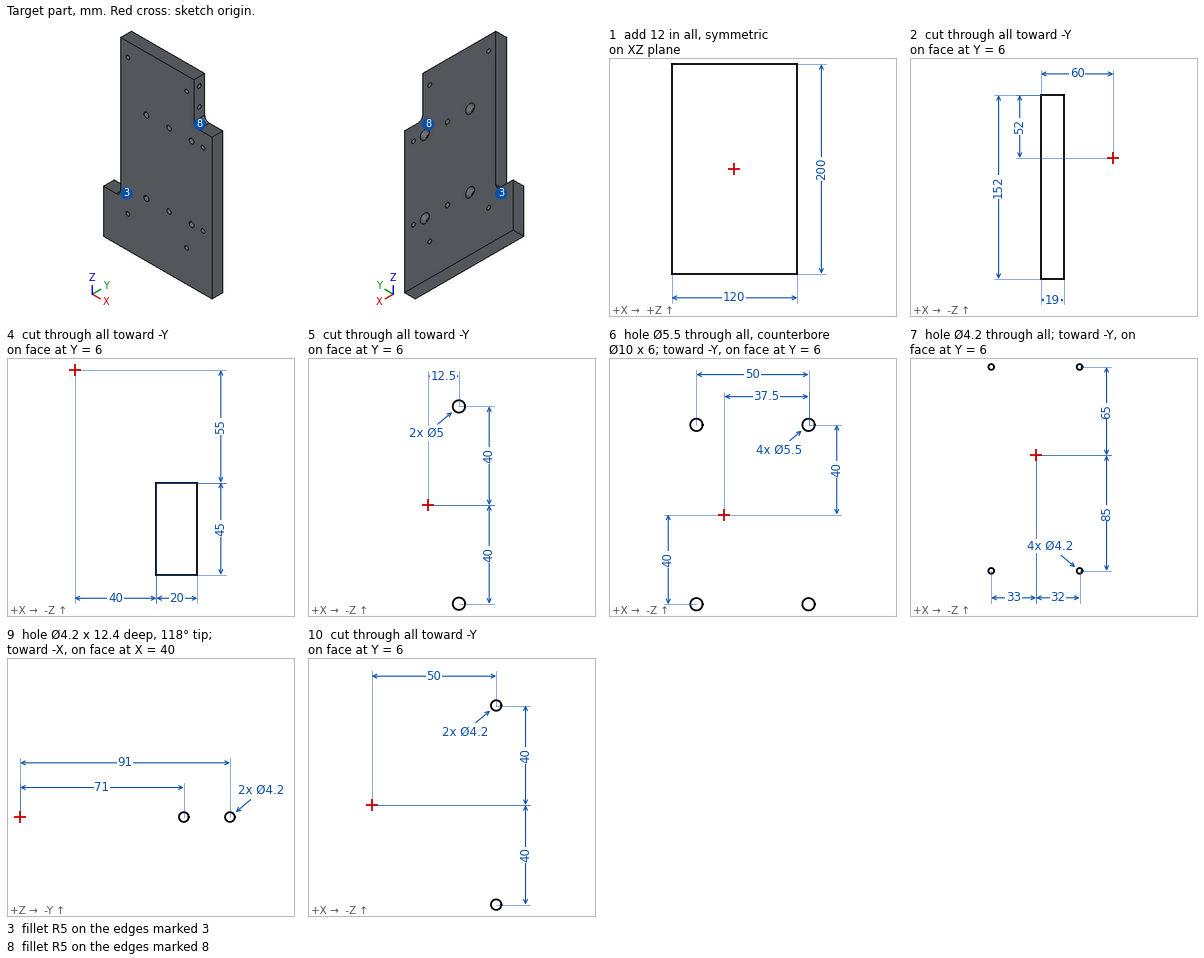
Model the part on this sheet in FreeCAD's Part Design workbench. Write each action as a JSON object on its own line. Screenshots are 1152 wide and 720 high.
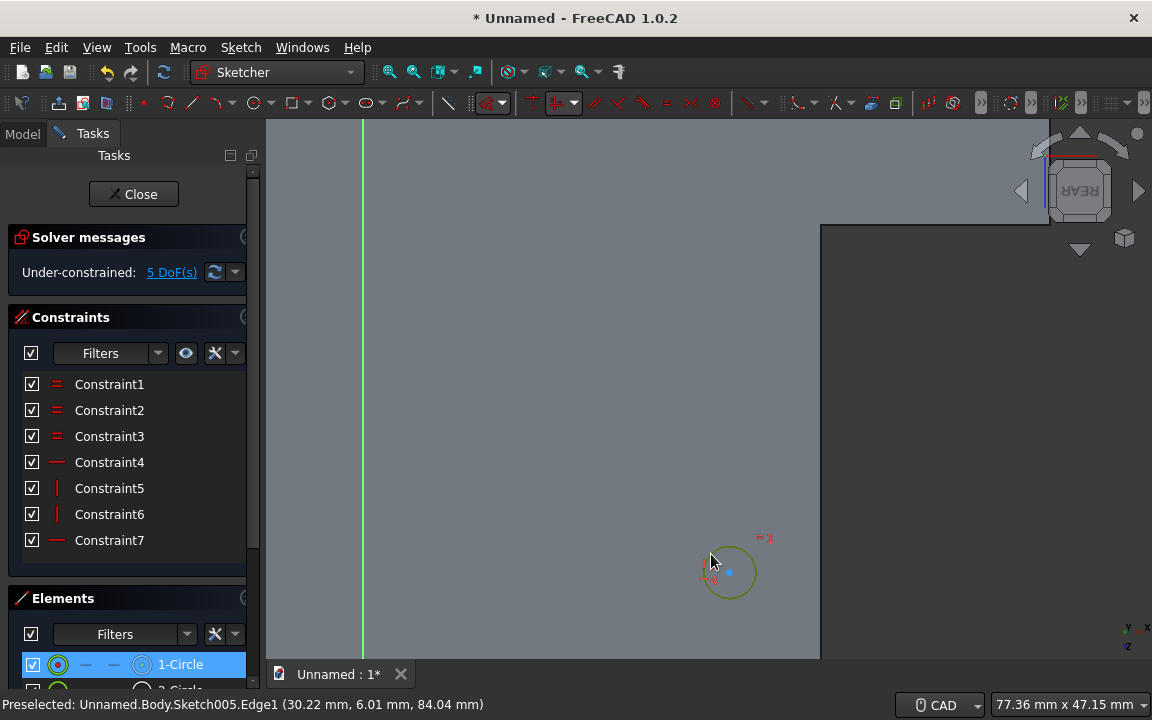
{"action": "left_click", "coordinate": [504, 104]}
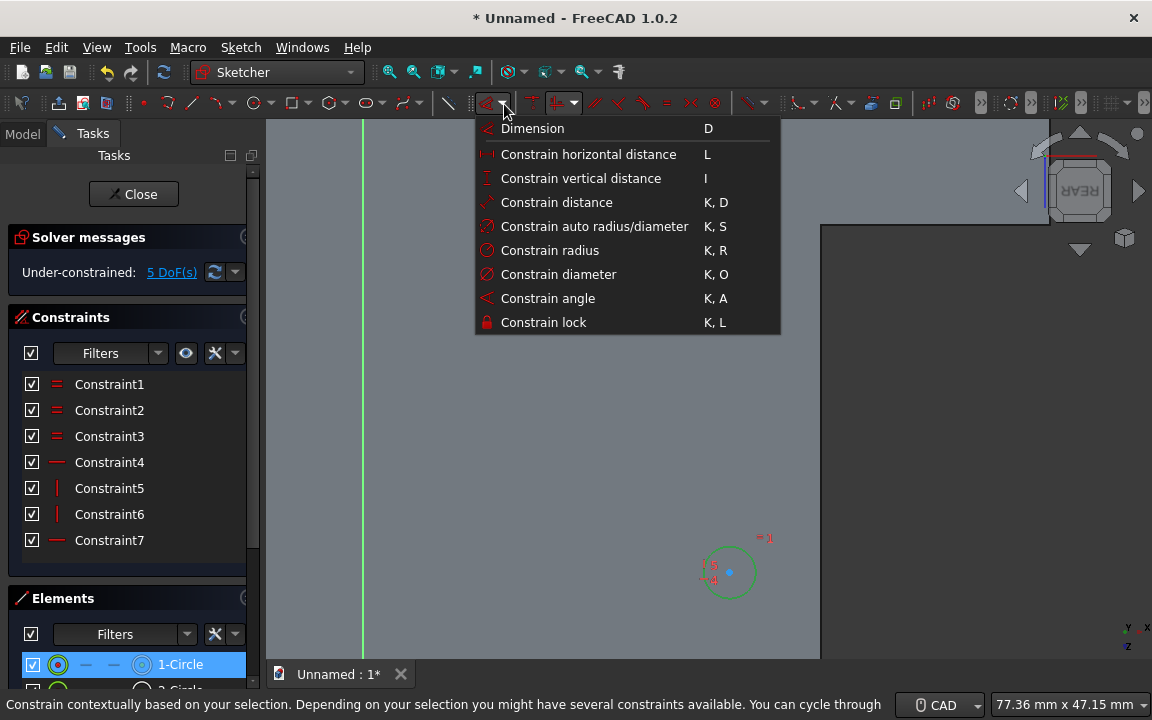
{"action": "left_click", "coordinate": [628, 274]}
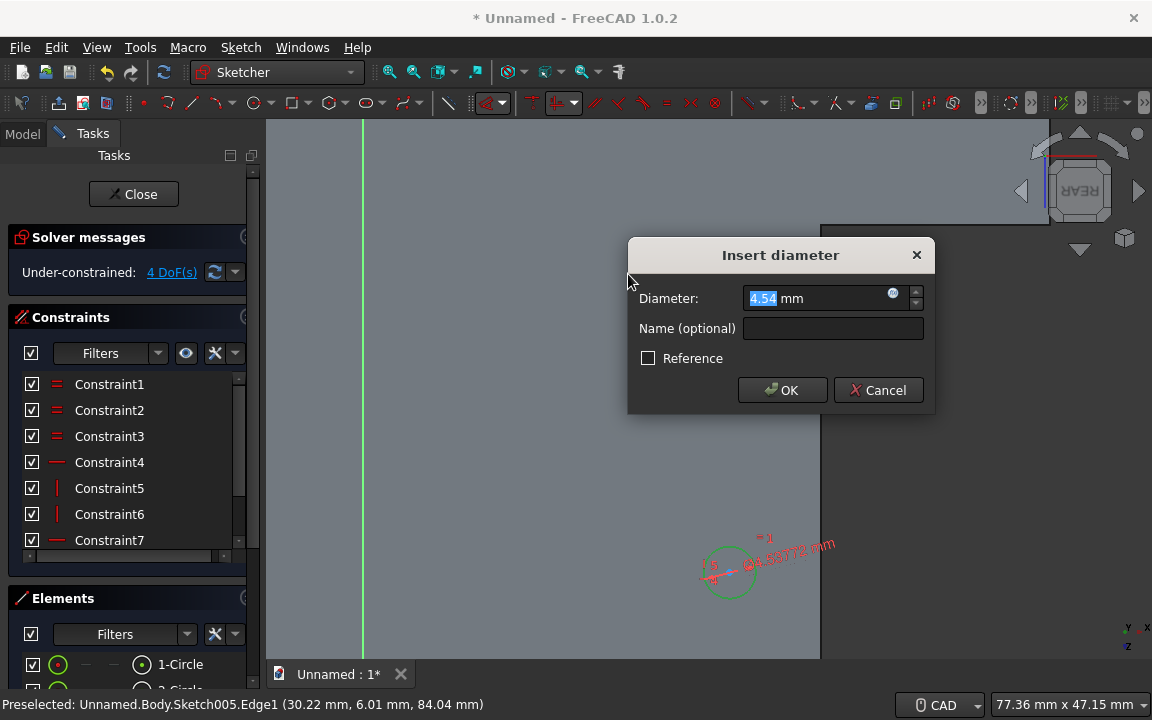
{"action": "type", "text": "4.2"}
{"action": "key", "text": "Return"}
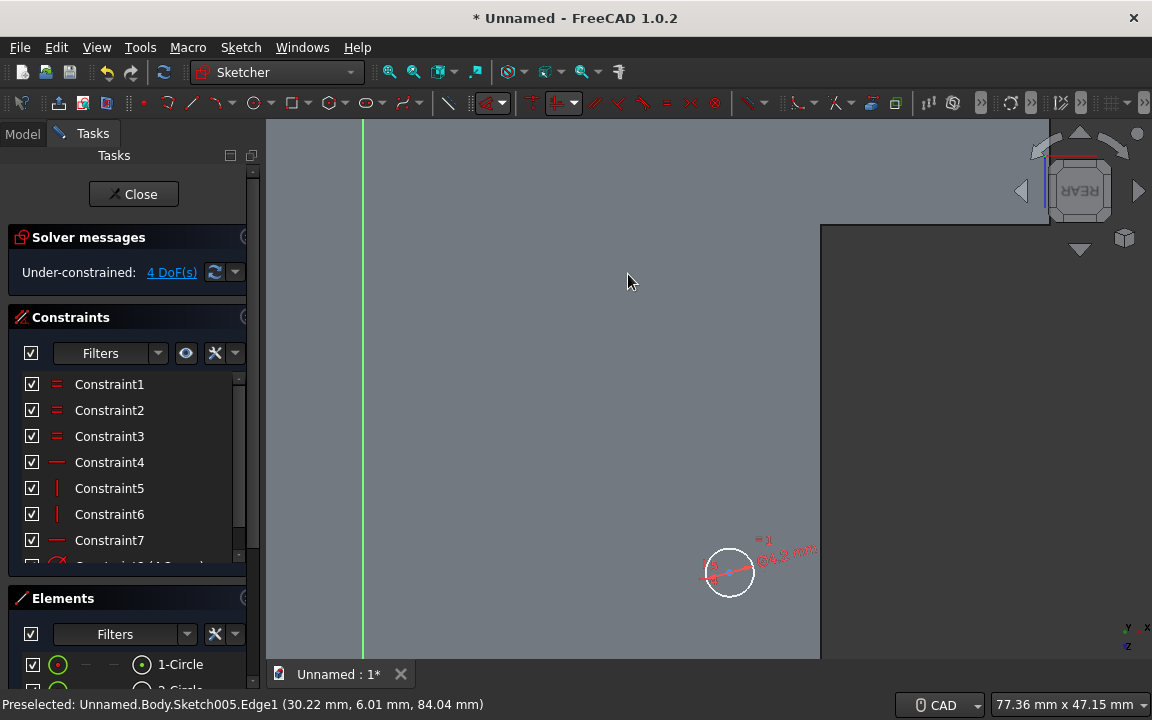
{"action": "scroll", "coordinate": [712, 561], "scroll_direction": "down", "scroll_amount": 8}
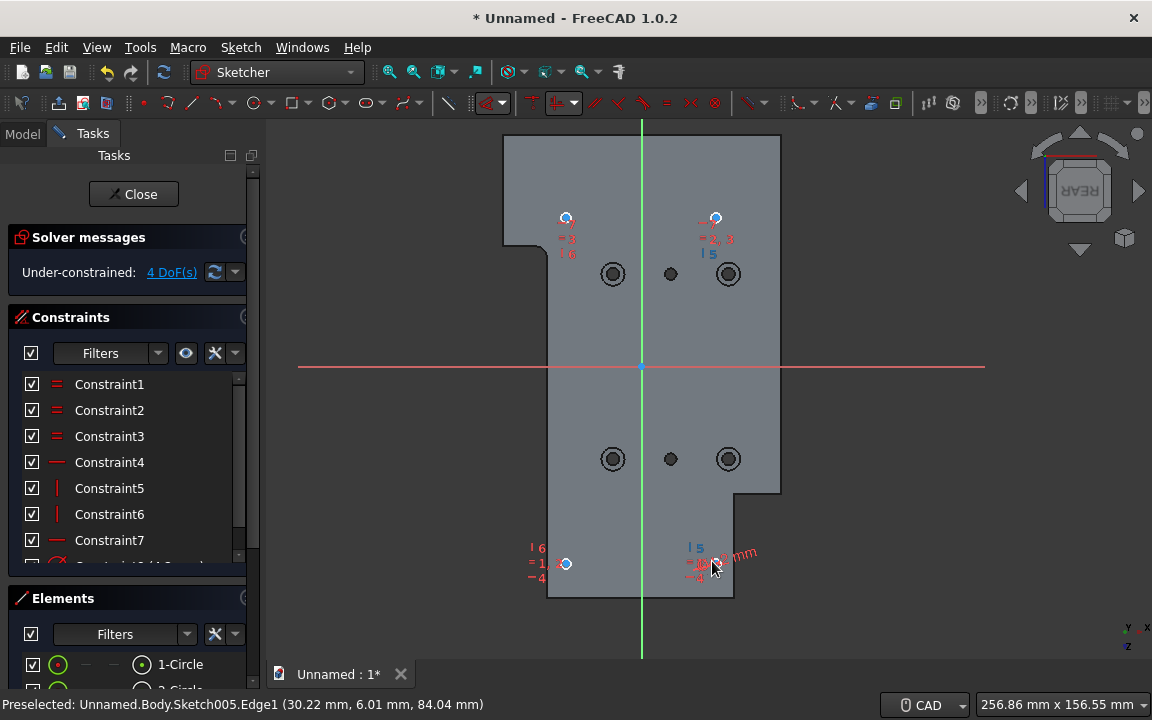
{"action": "left_click", "coordinate": [716, 564]}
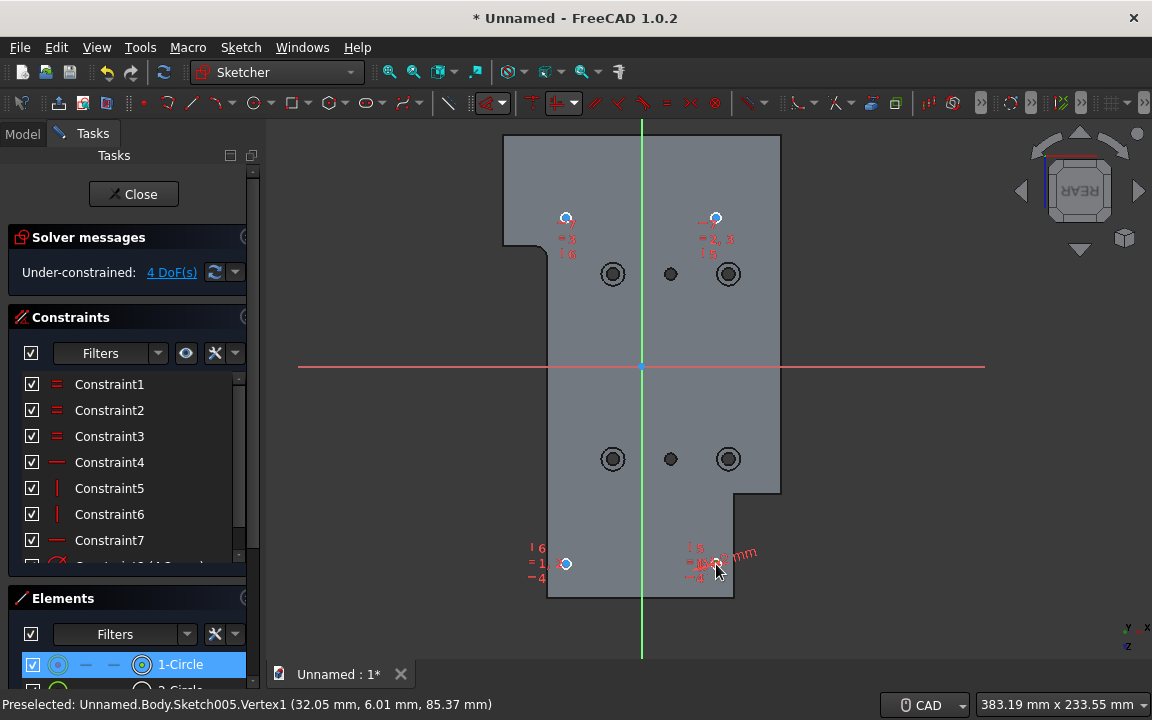
{"action": "left_click", "coordinate": [504, 104]}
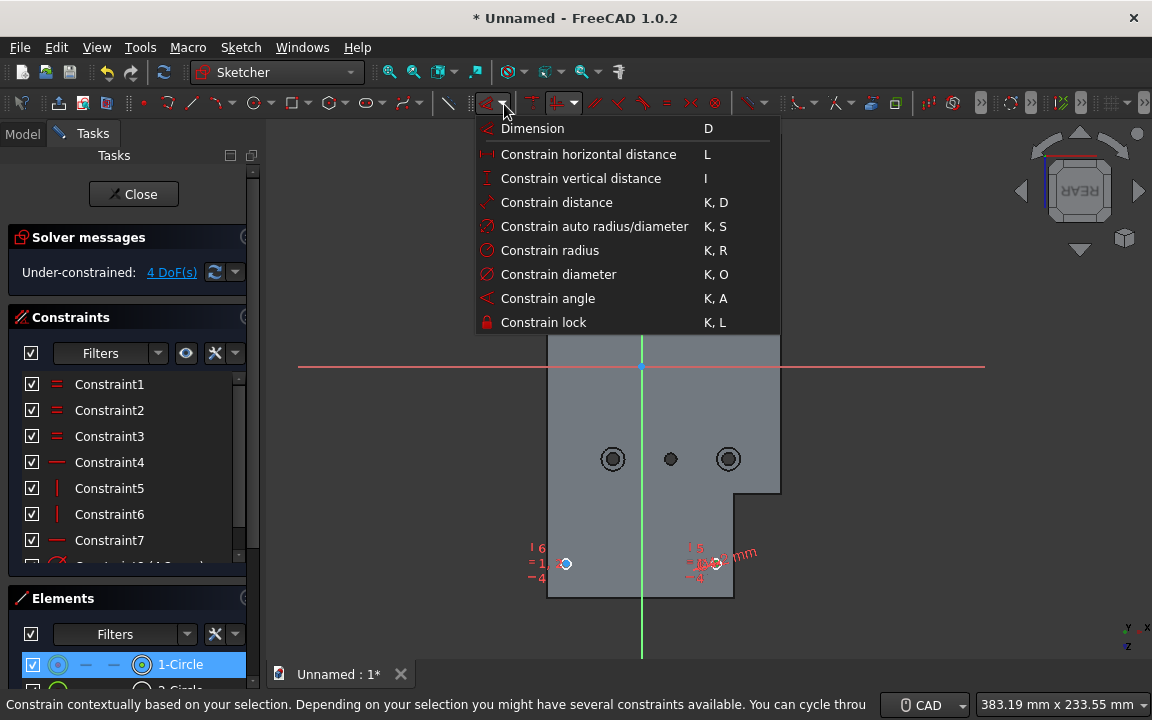
{"action": "left_click", "coordinate": [628, 154]}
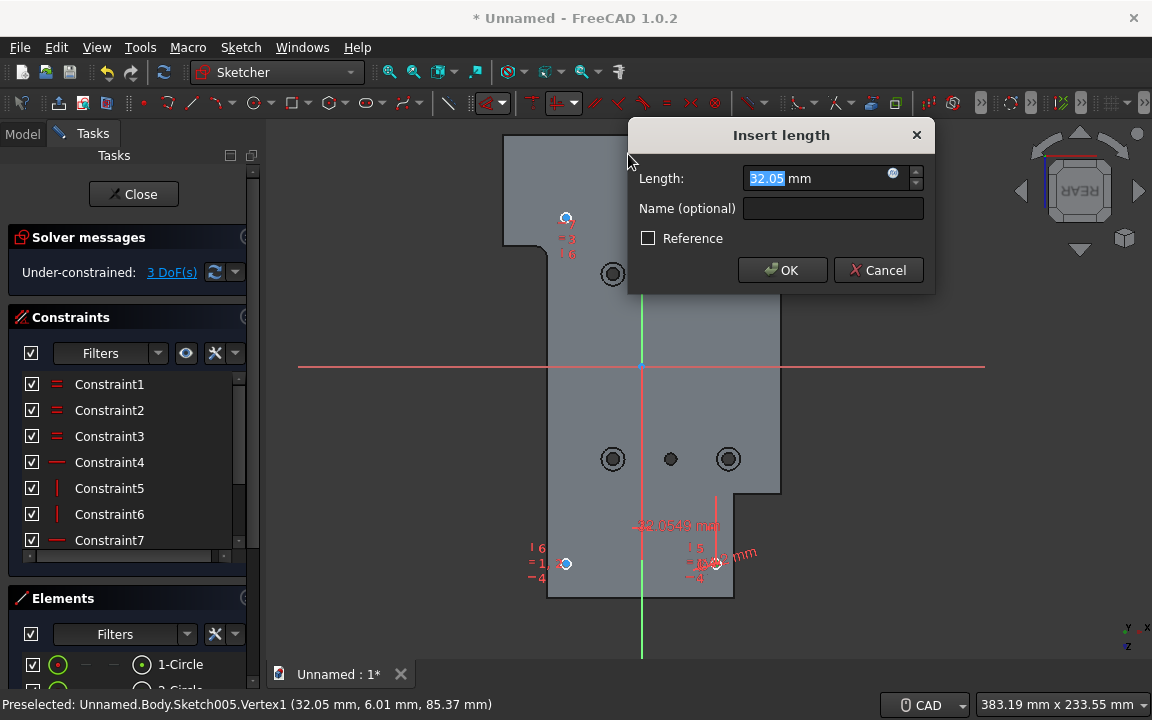
{"action": "type", "text": "32"}
{"action": "key", "text": "Return"}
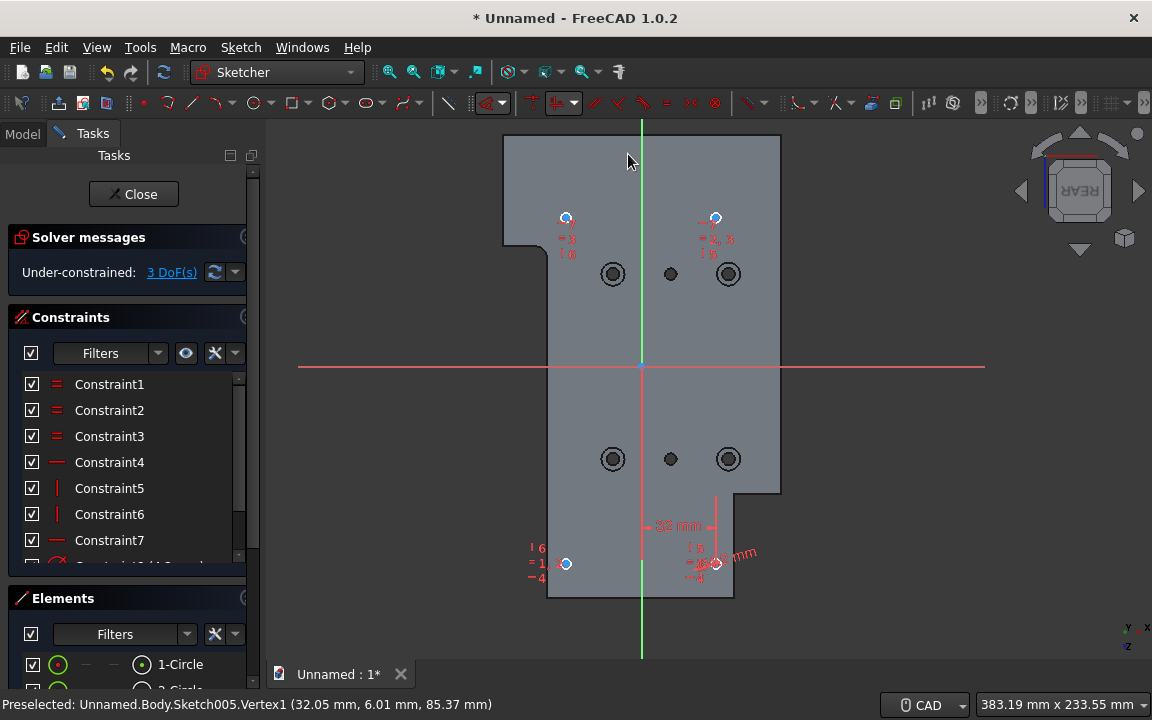
{"action": "left_click", "coordinate": [716, 564]}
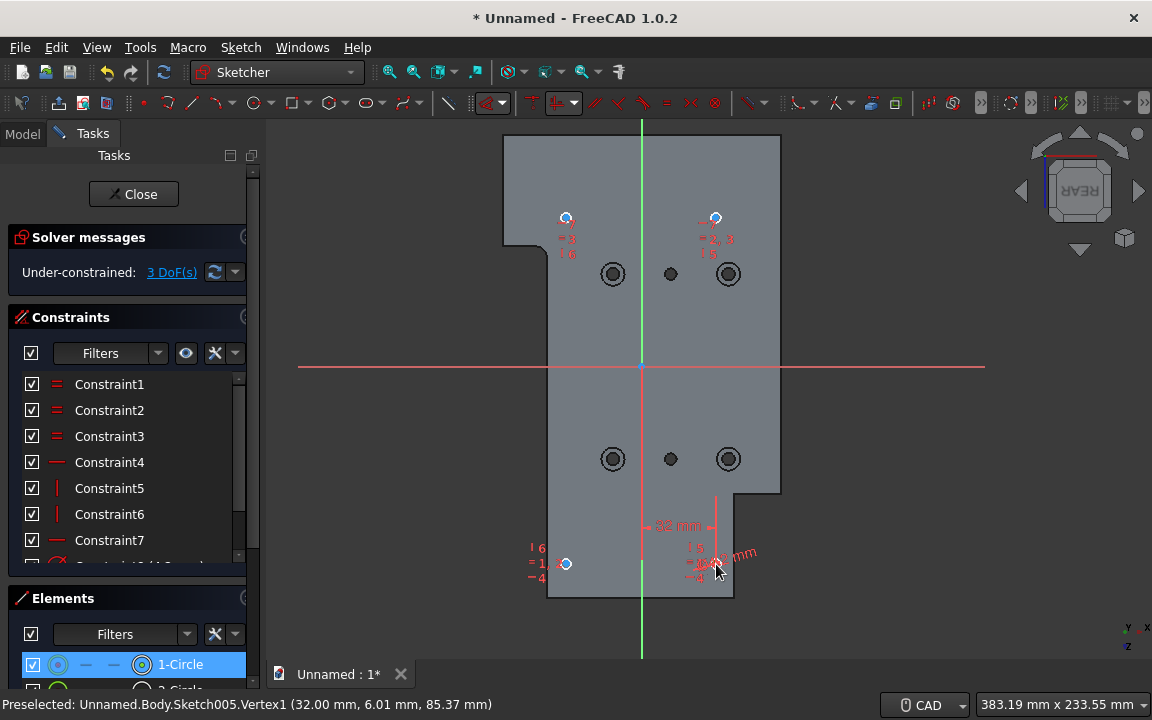
{"action": "left_click", "coordinate": [504, 104]}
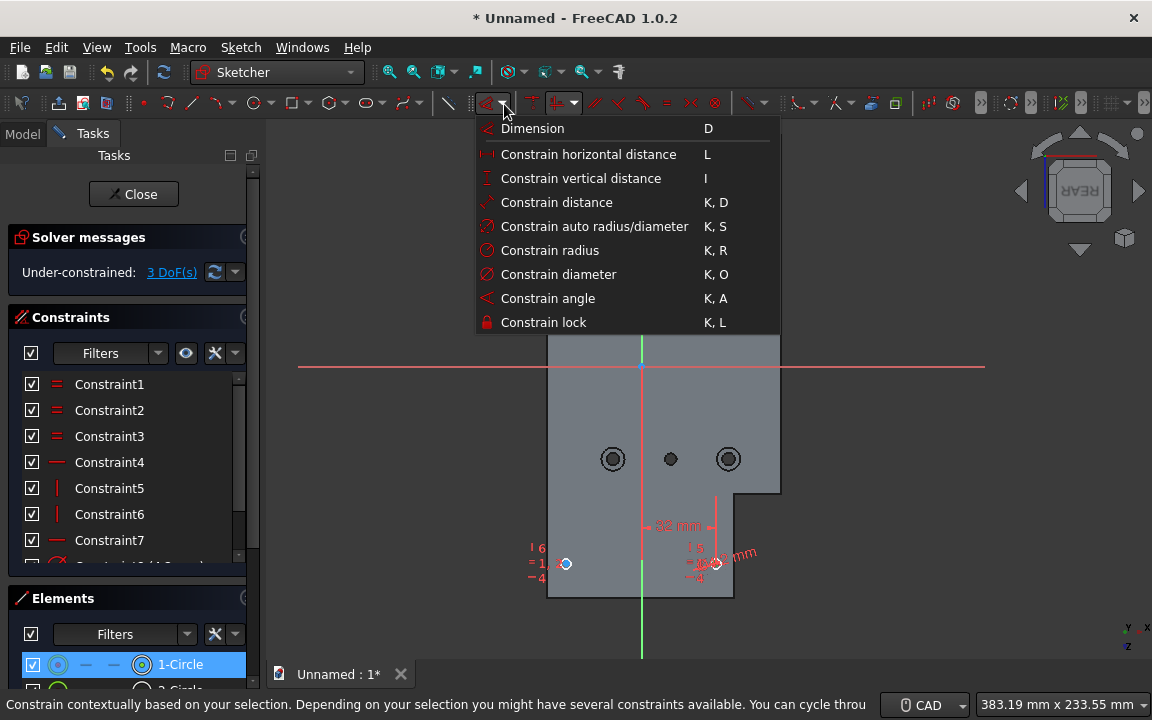
{"action": "left_click", "coordinate": [628, 178]}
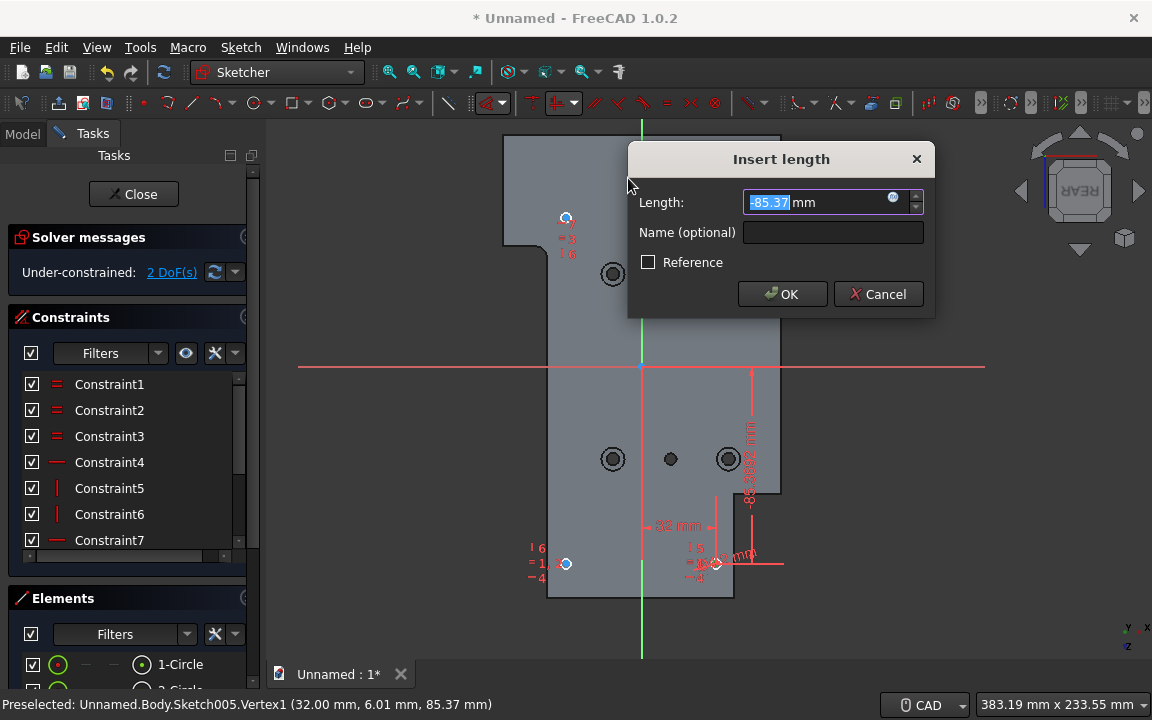
{"action": "type", "text": "-85"}
{"action": "key", "text": "Return"}